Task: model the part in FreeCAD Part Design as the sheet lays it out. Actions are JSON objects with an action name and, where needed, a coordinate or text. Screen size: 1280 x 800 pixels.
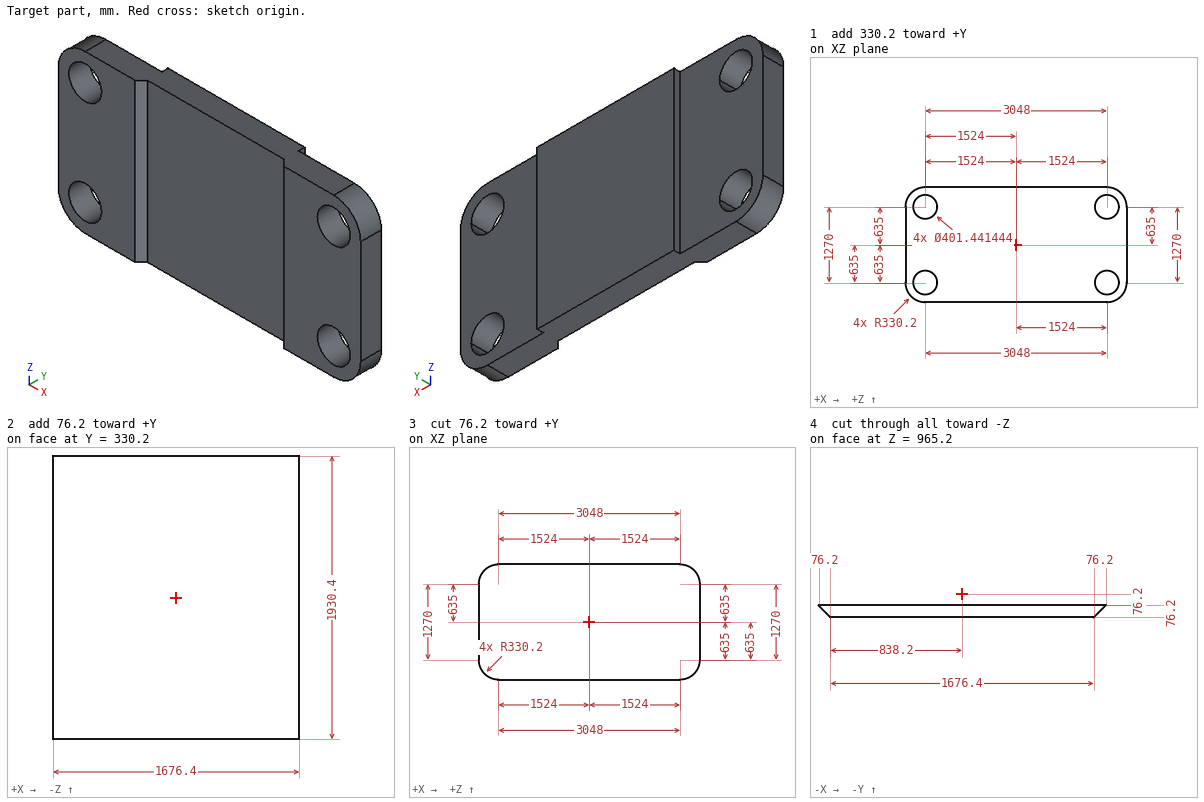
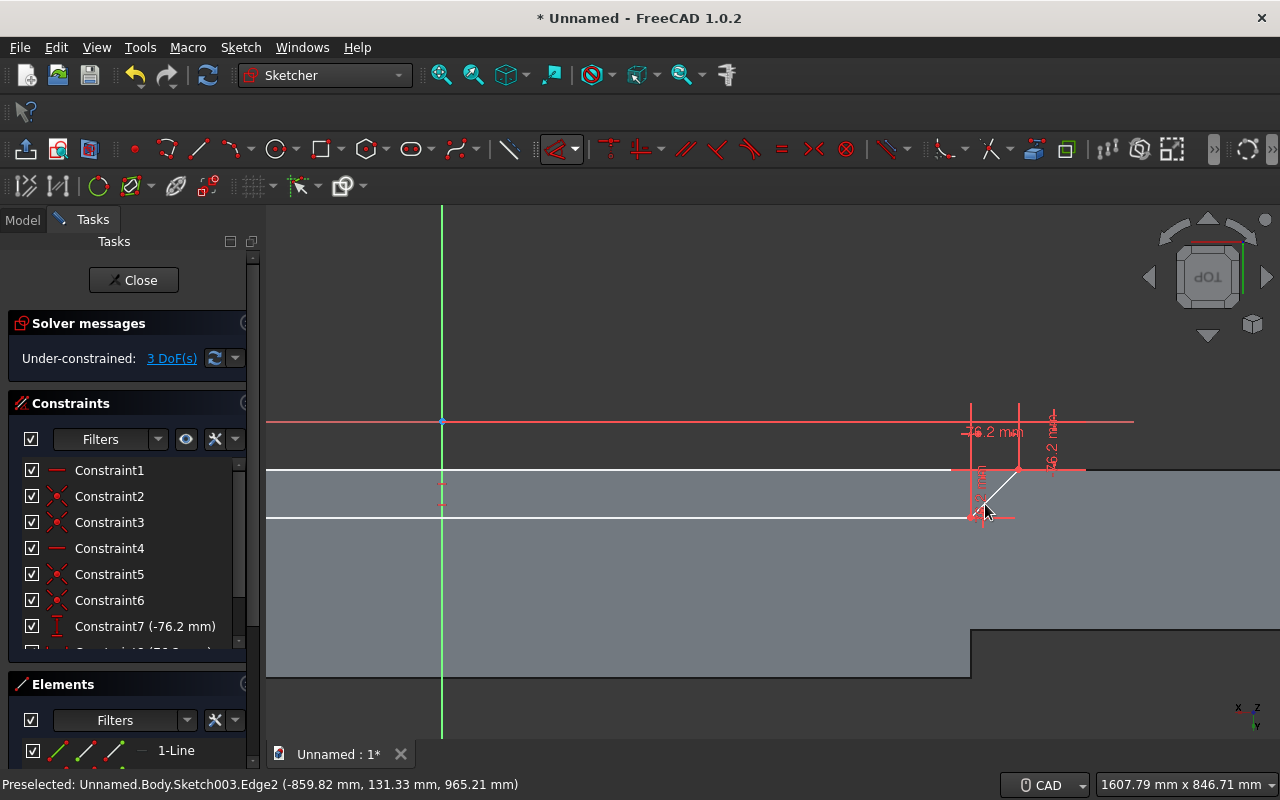
{"action": "scroll", "coordinate": [1023, 475], "scroll_direction": "down", "scroll_amount": 3}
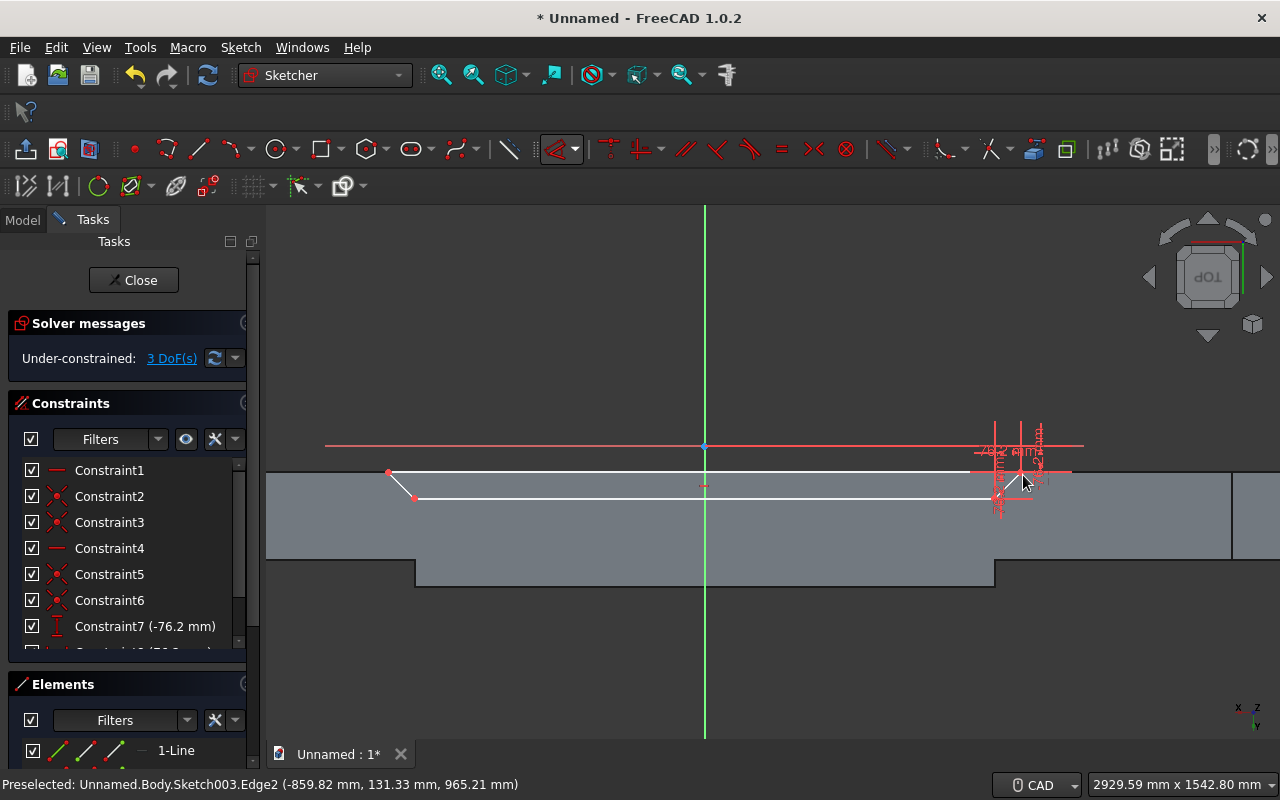
{"action": "scroll", "coordinate": [396, 480], "scroll_direction": "up", "scroll_amount": 3}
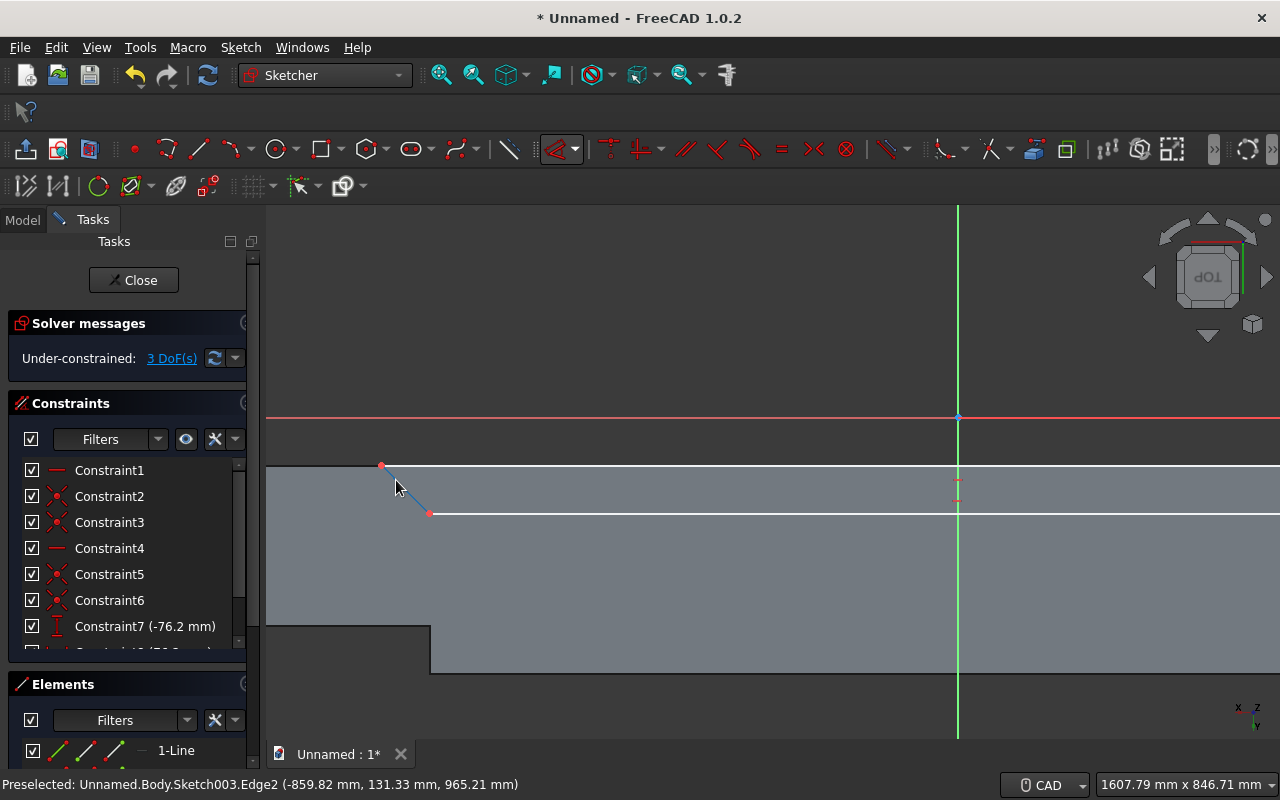
{"action": "left_click", "coordinate": [396, 480]}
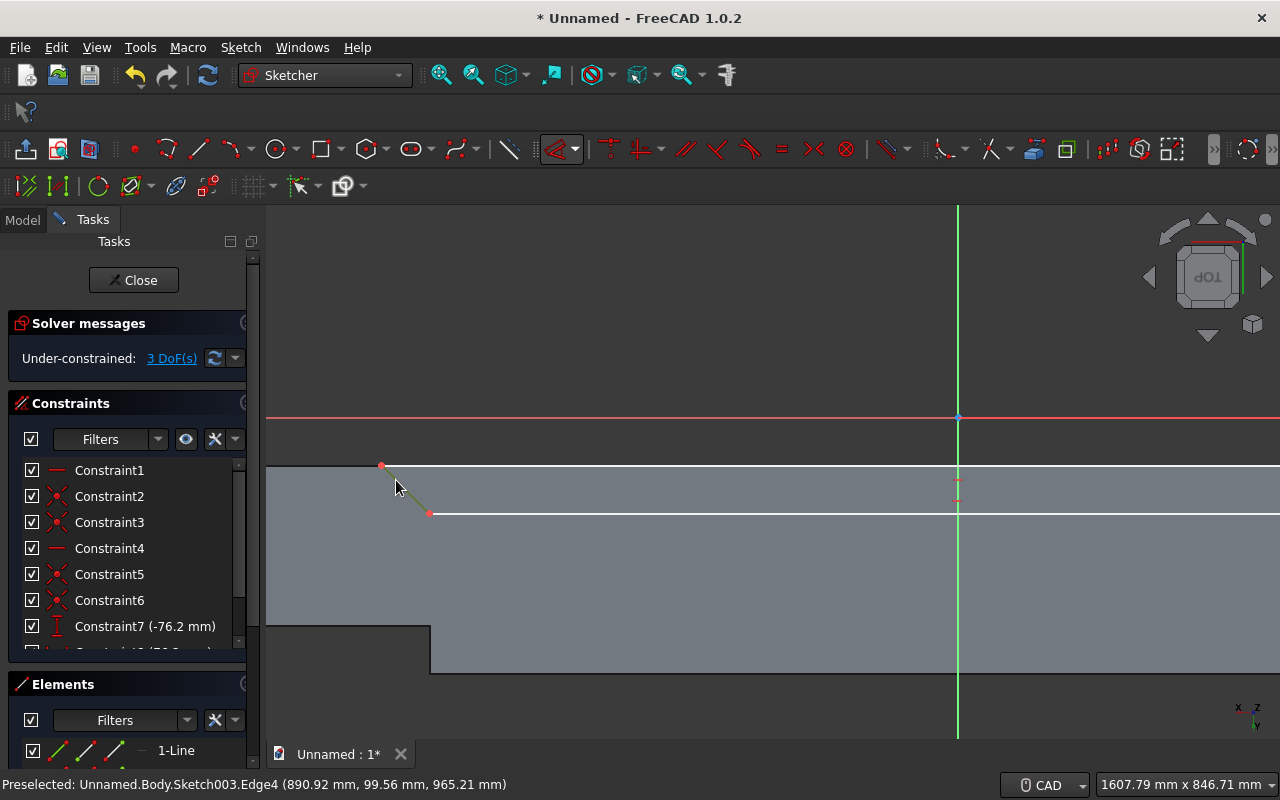
{"action": "key", "text": "l"}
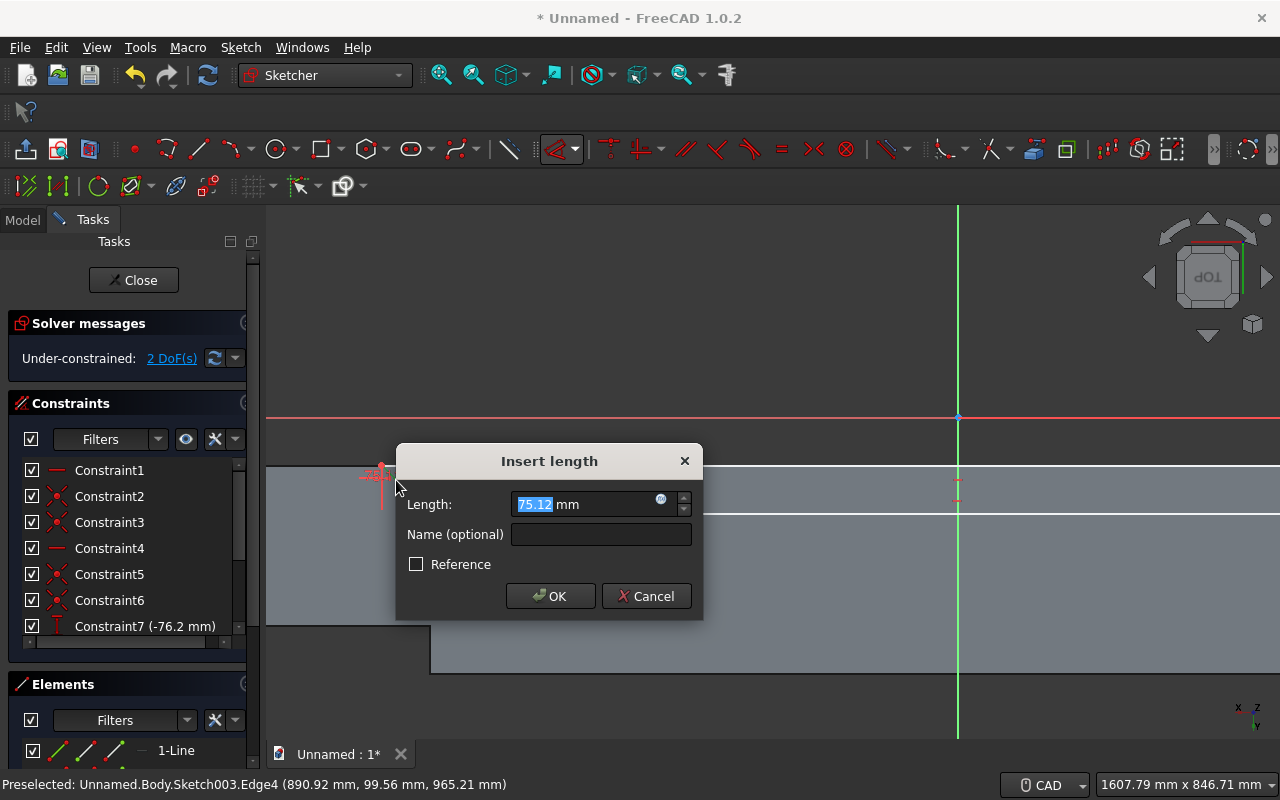
{"action": "type", "text": "76.2"}
{"action": "key", "text": "Return"}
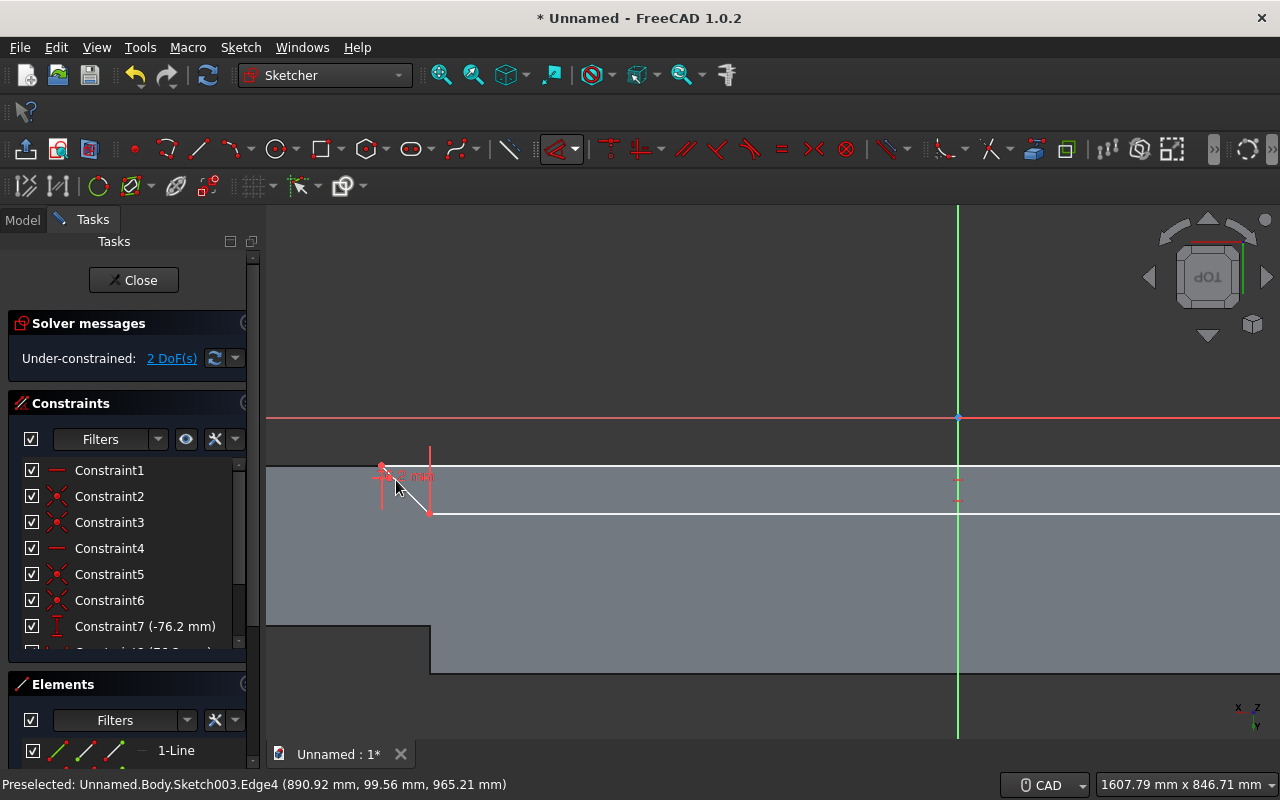
{"action": "left_click", "coordinate": [747, 514]}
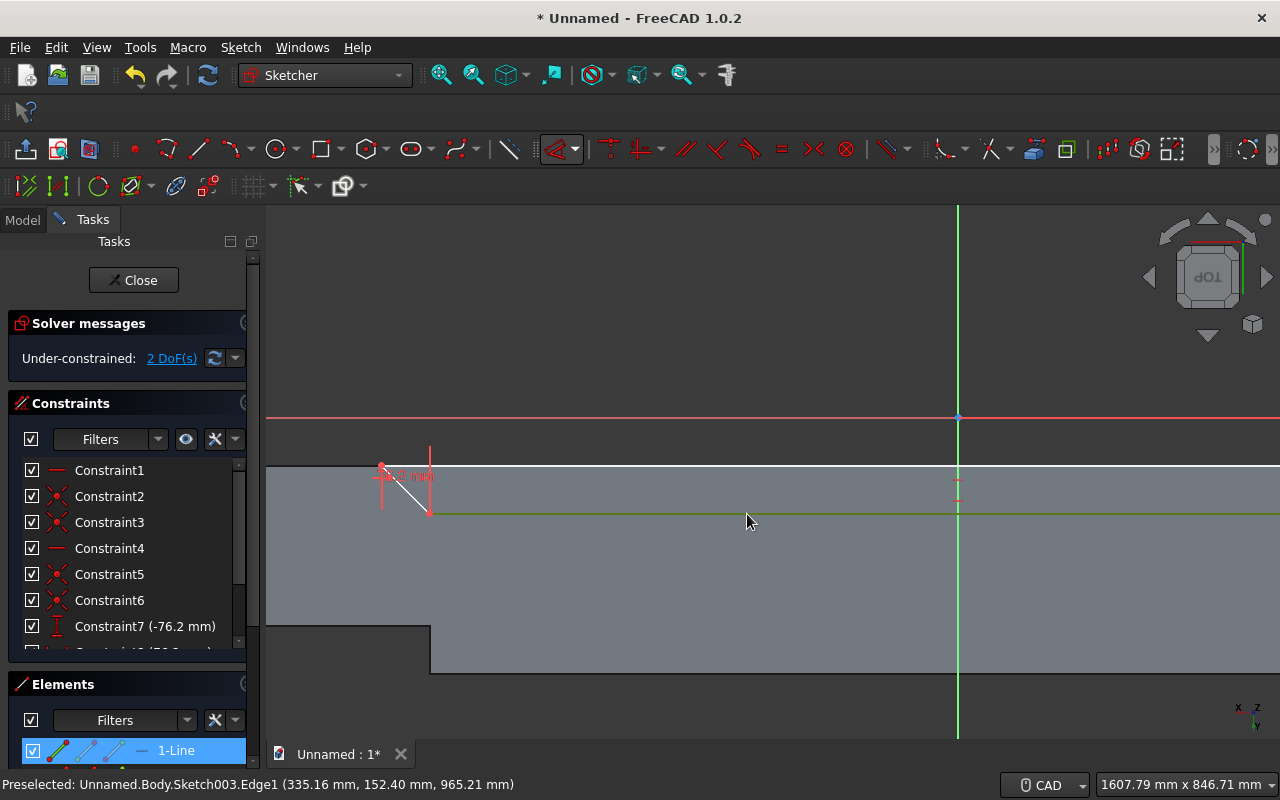
{"action": "key", "text": "l"}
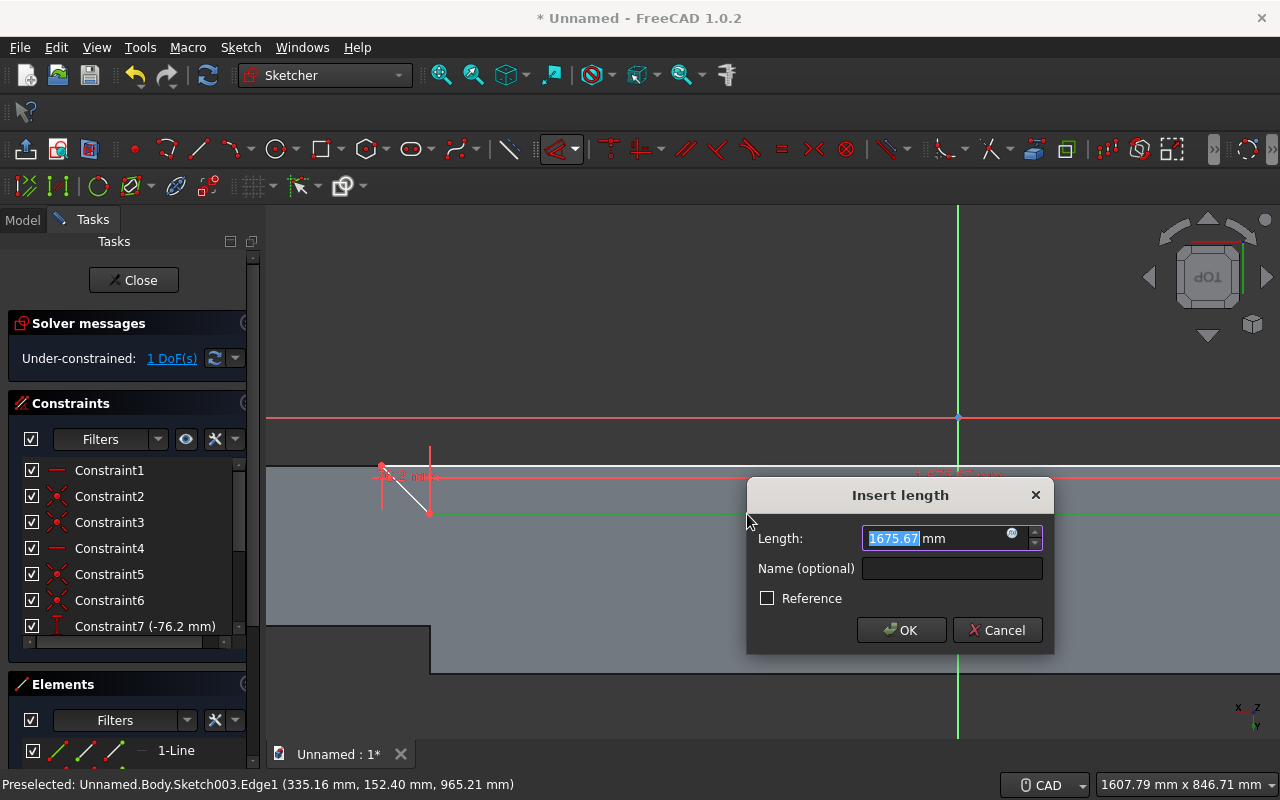
{"action": "type", "text": "1676.4"}
{"action": "key", "text": "Return"}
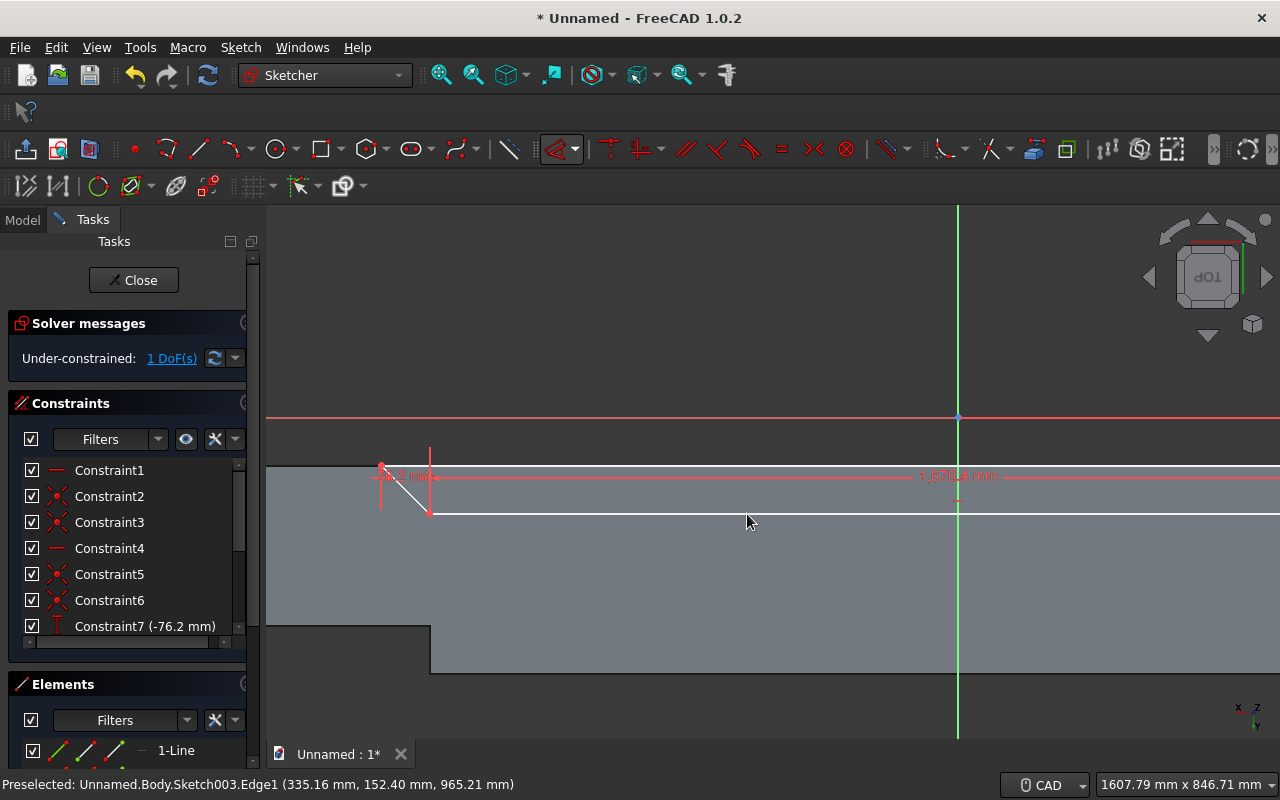
{"action": "left_click", "coordinate": [430, 514]}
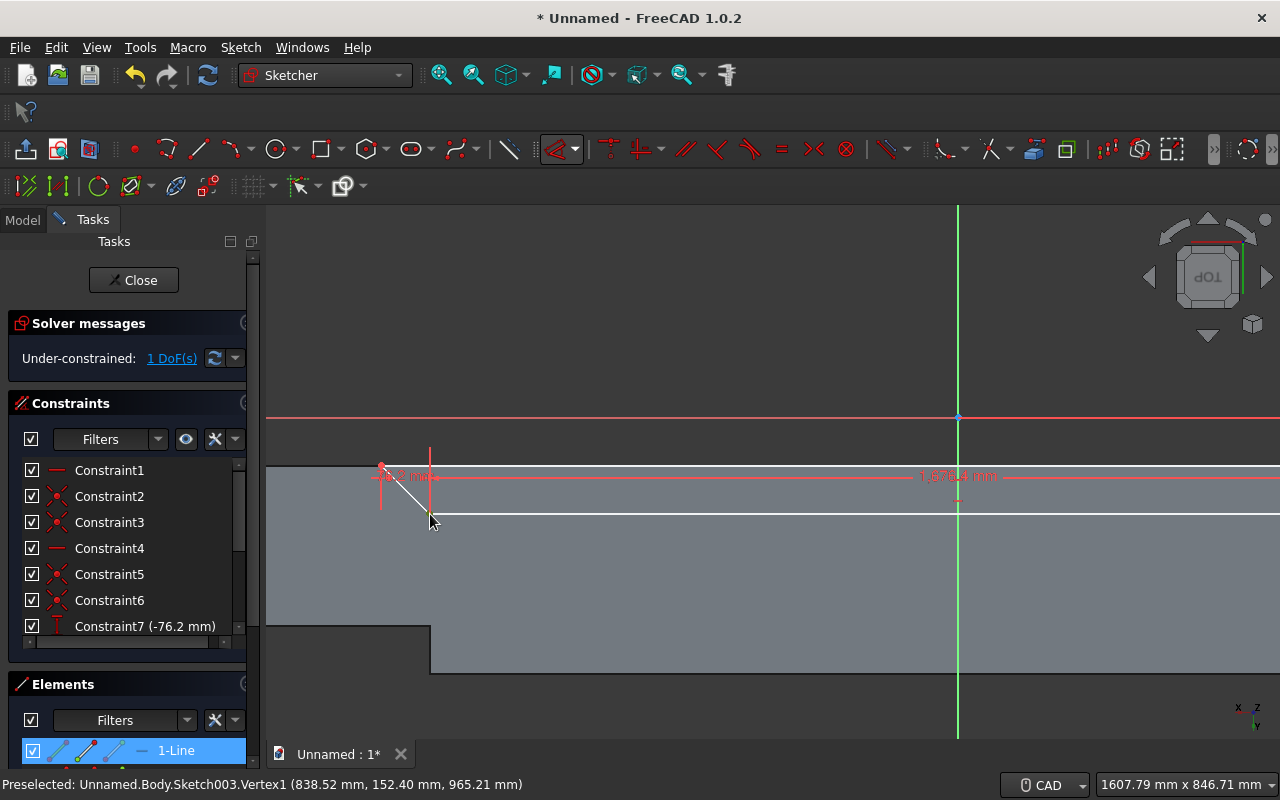
{"action": "key", "text": "l"}